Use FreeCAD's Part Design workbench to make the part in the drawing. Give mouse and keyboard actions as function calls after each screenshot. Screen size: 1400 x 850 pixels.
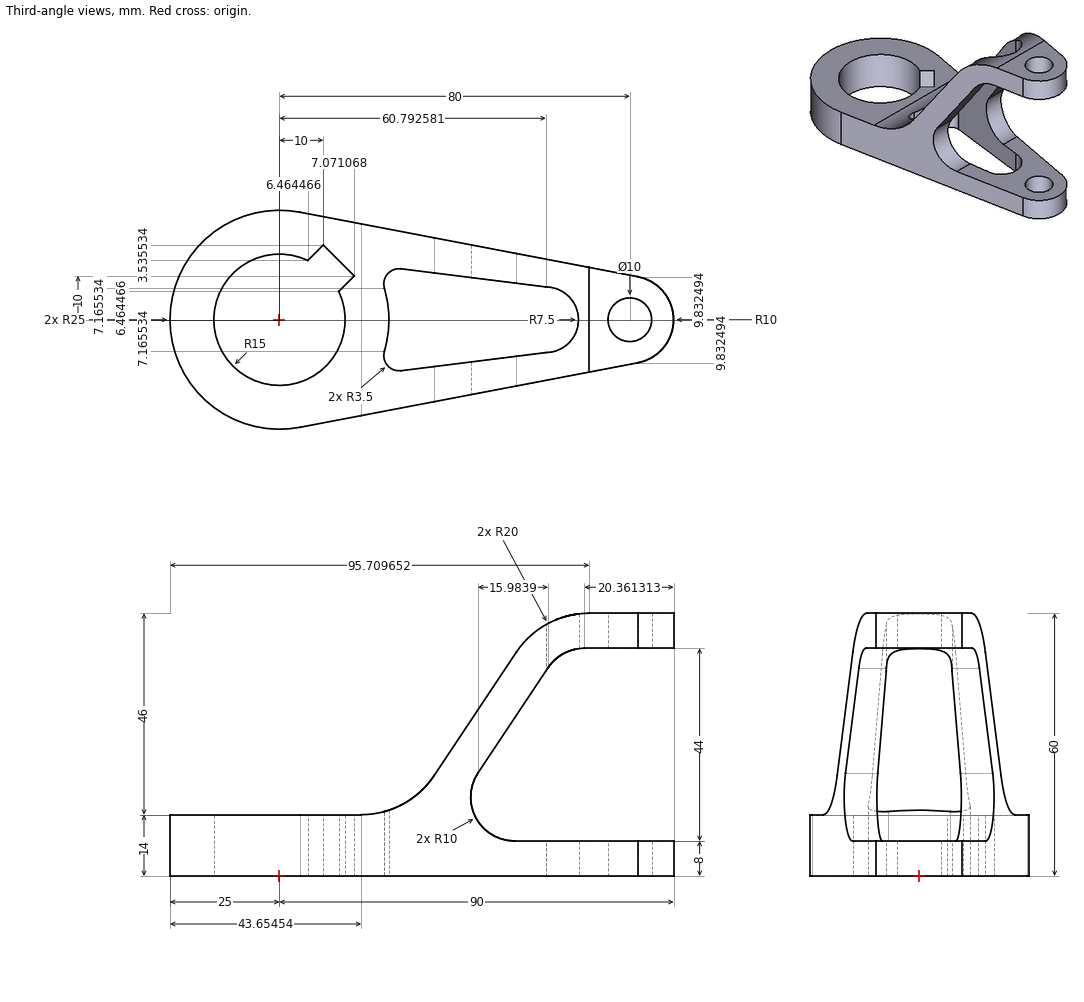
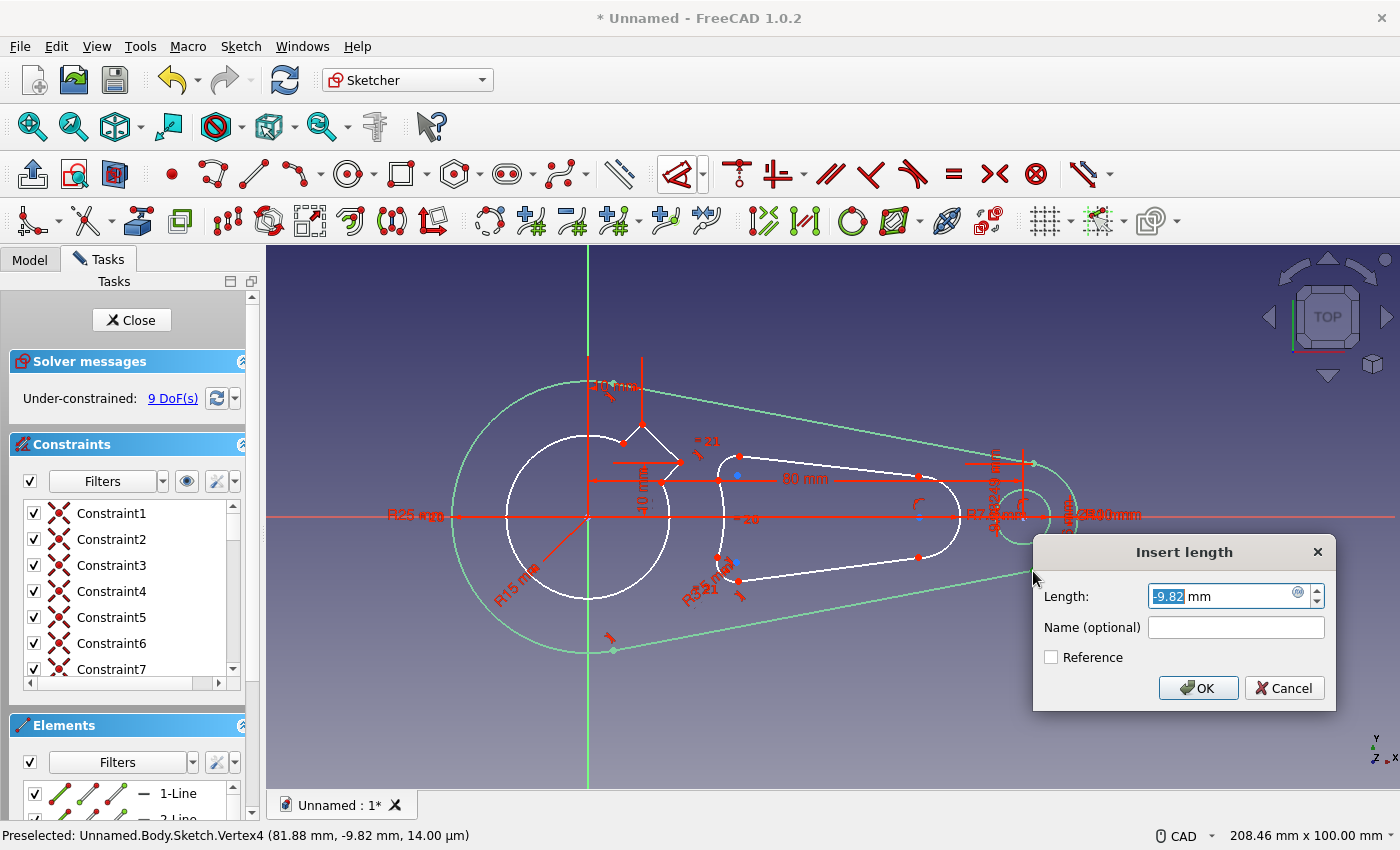
text(-9.832494)
key(Return)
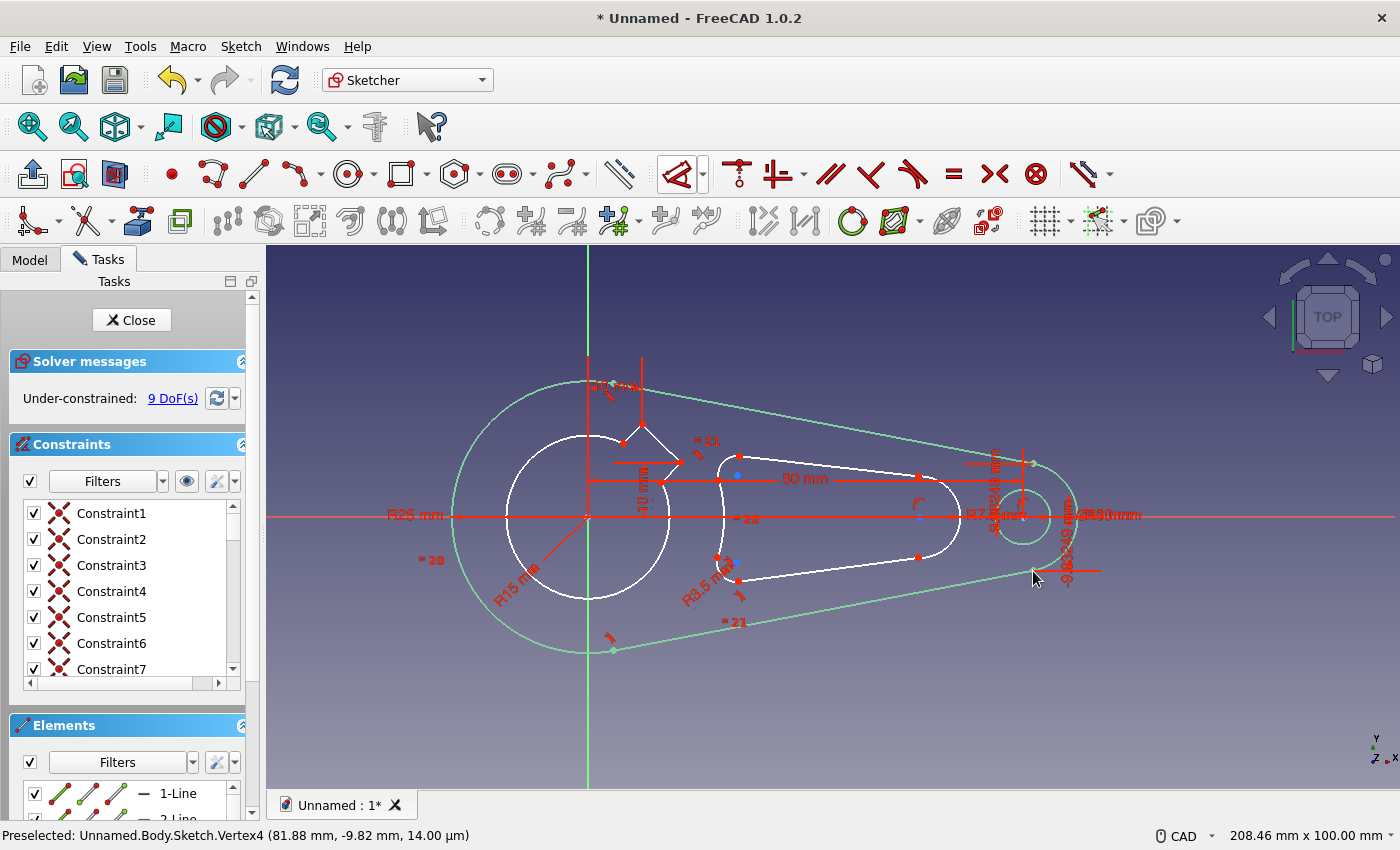
click(718, 557)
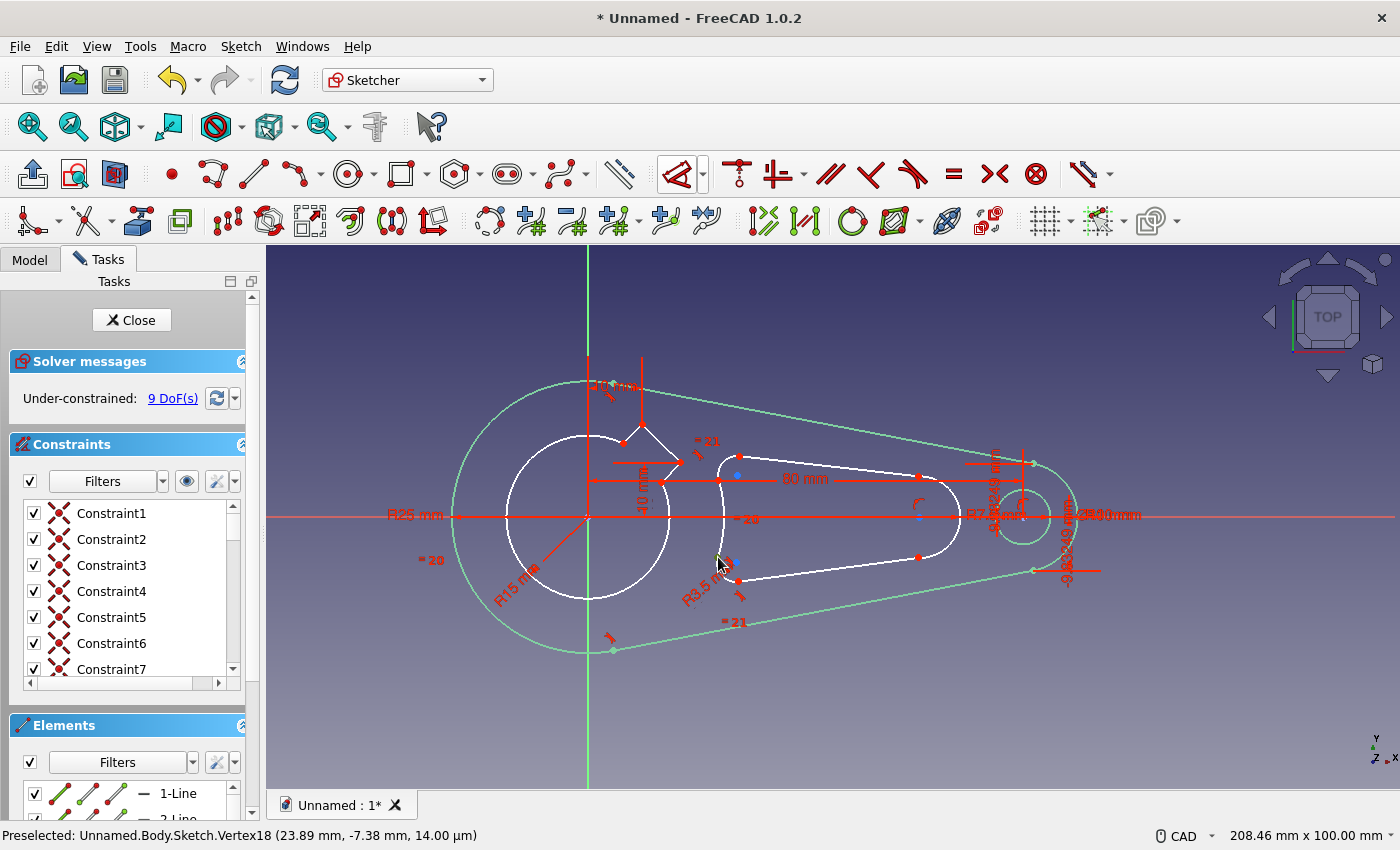
click(702, 174)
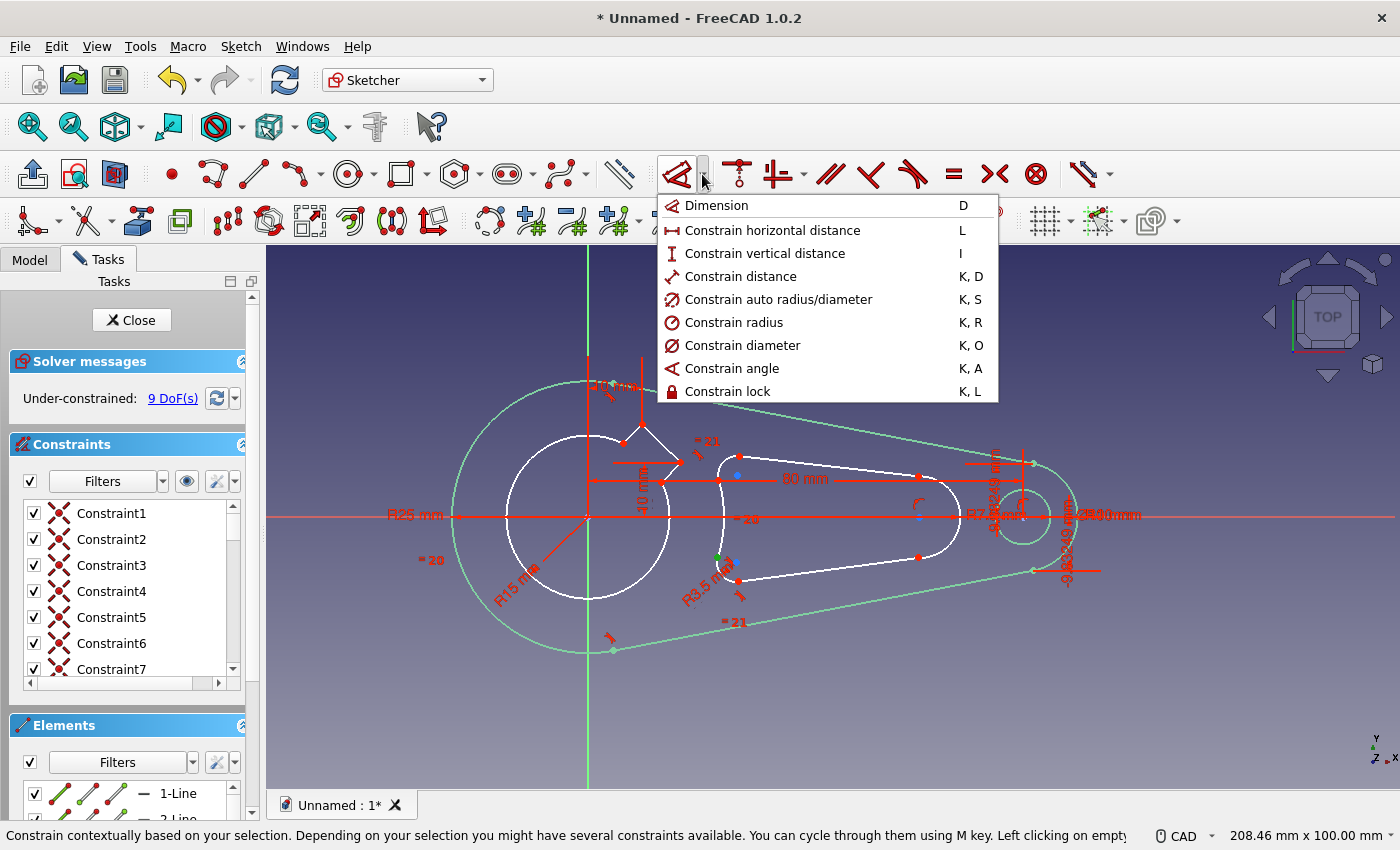
click(828, 254)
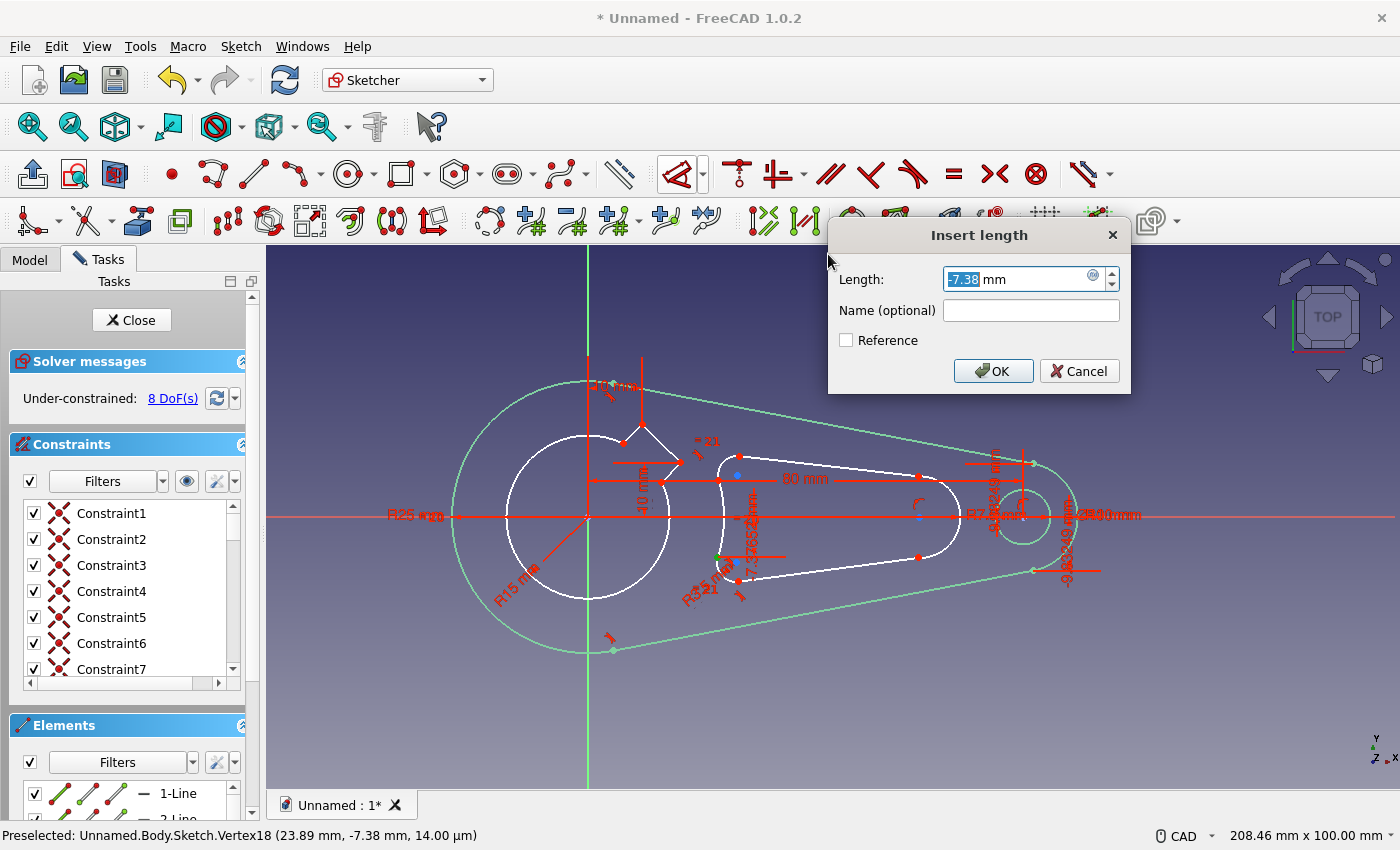
text(-7.165534)
key(Return)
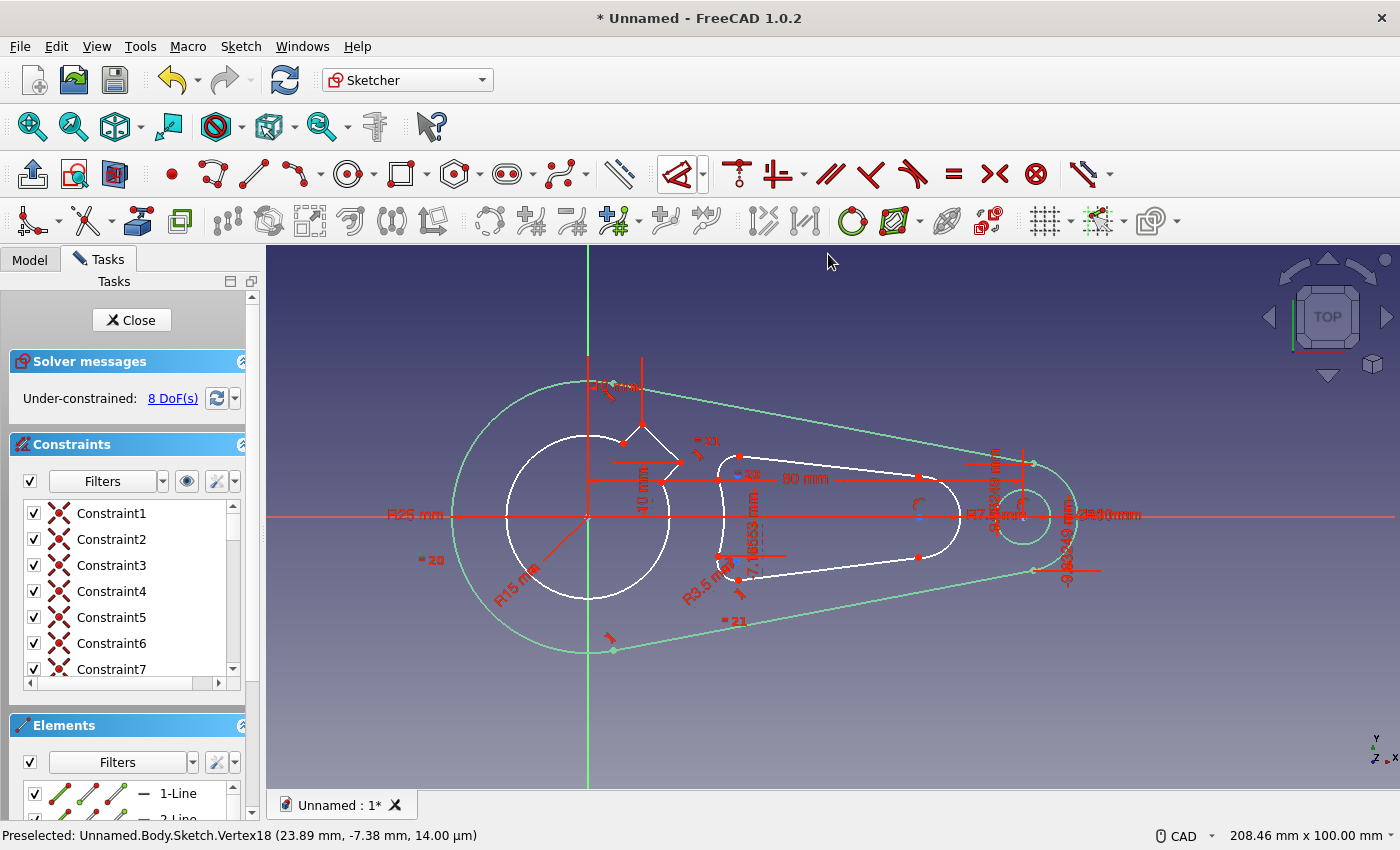
click(719, 480)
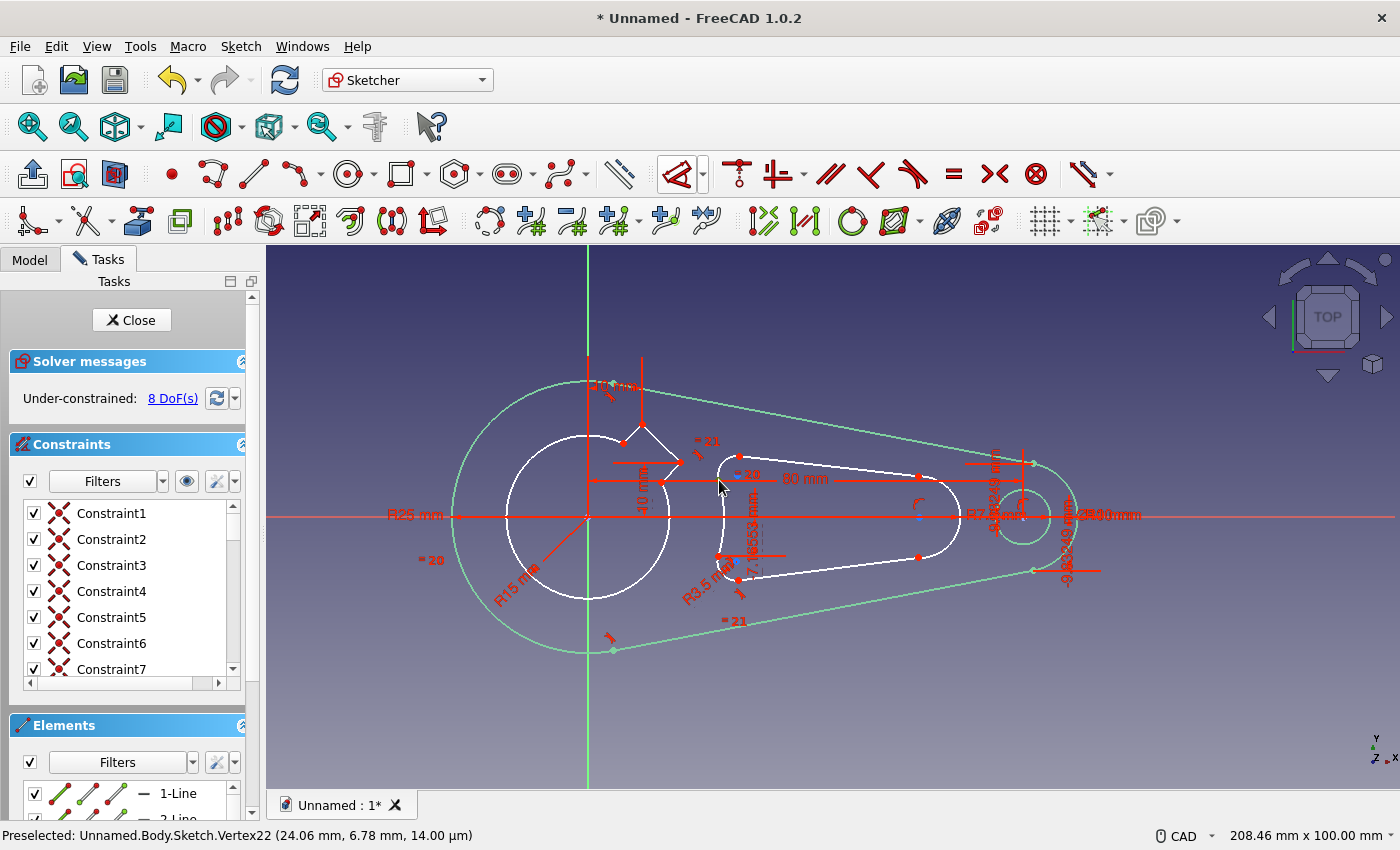
click(702, 174)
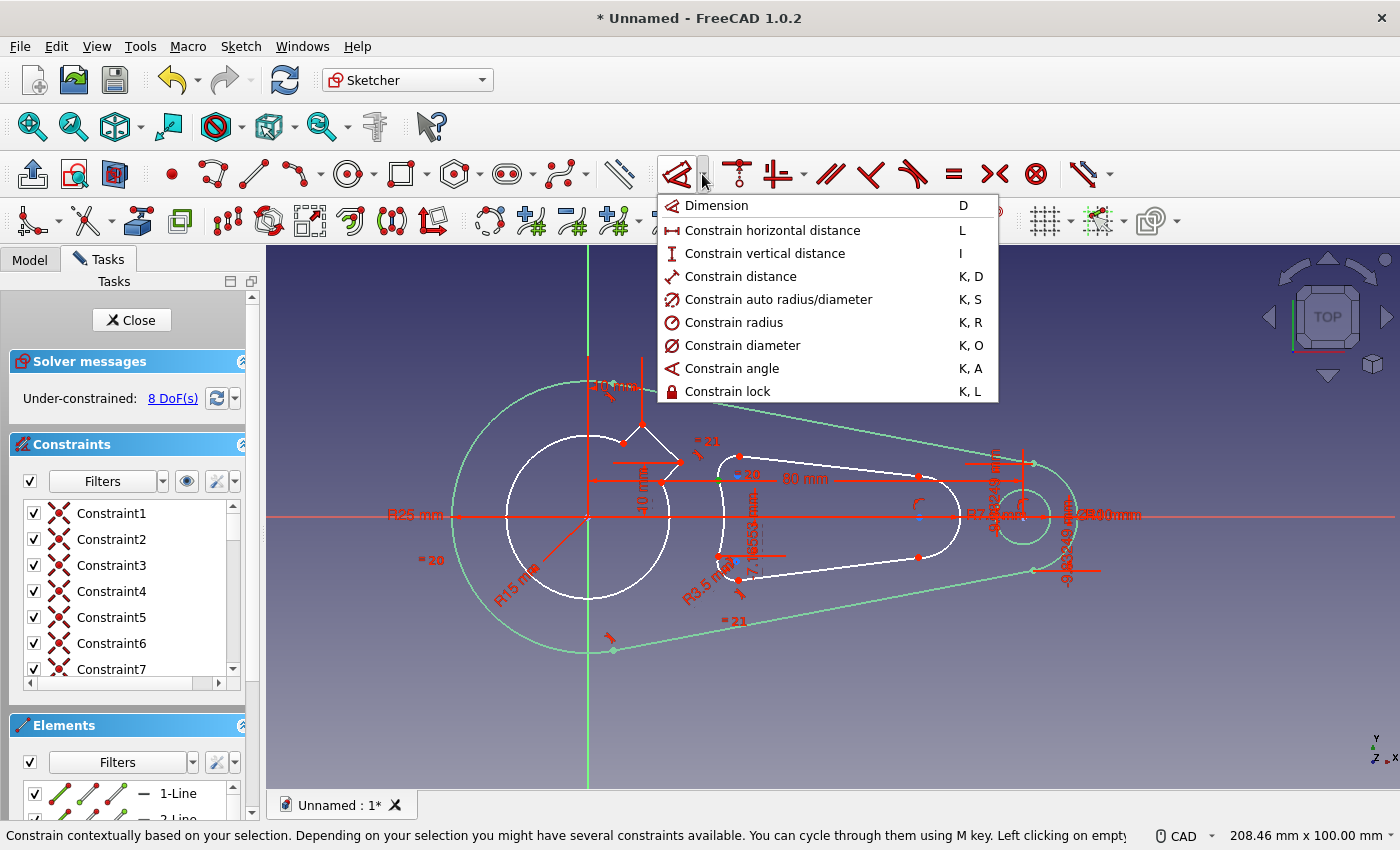
click(828, 254)